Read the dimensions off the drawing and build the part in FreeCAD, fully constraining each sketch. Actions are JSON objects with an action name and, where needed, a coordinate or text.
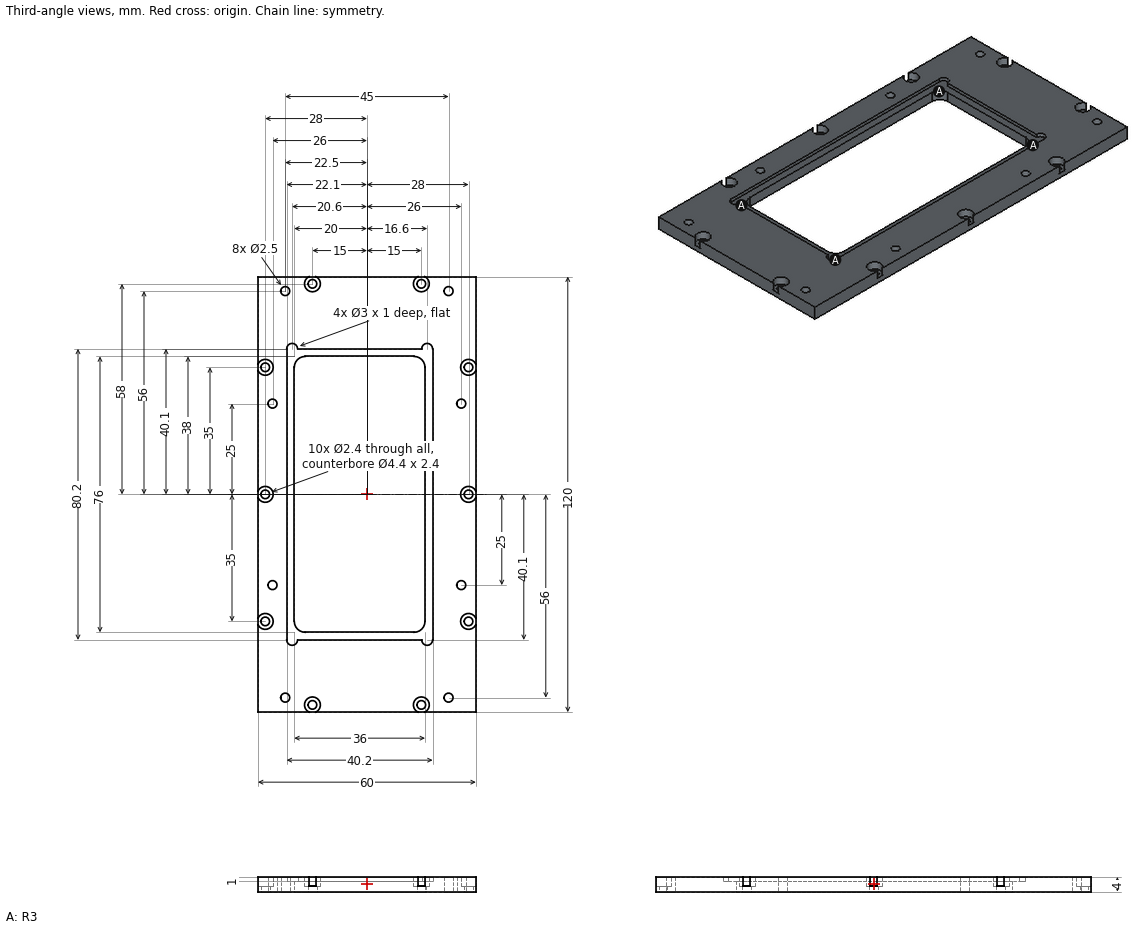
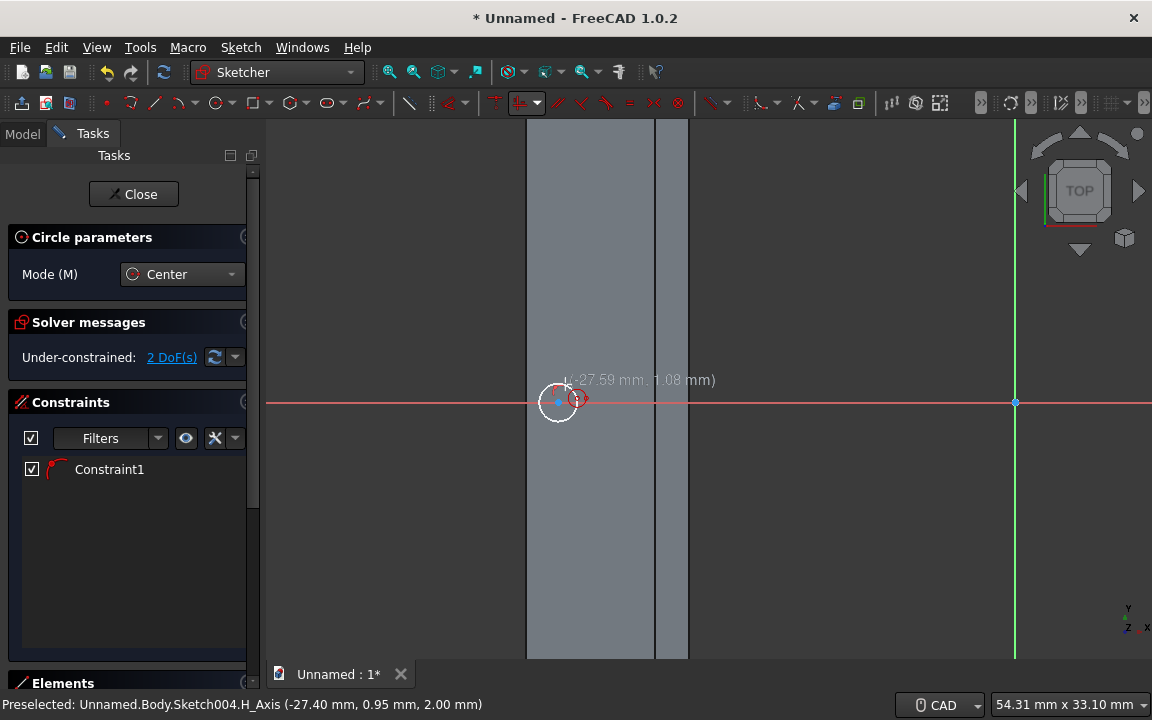
{"action": "scroll", "coordinate": [566, 386], "scroll_direction": "down", "scroll_amount": 9}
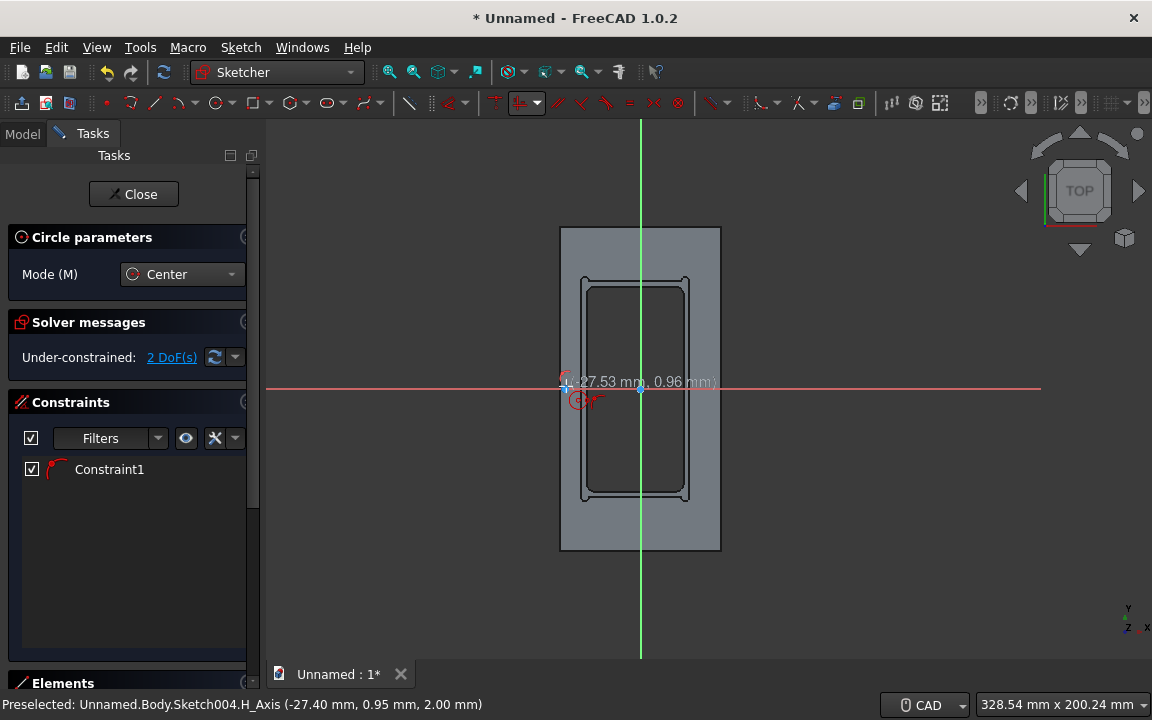
{"action": "scroll", "coordinate": [716, 389], "scroll_direction": "up", "scroll_amount": 10}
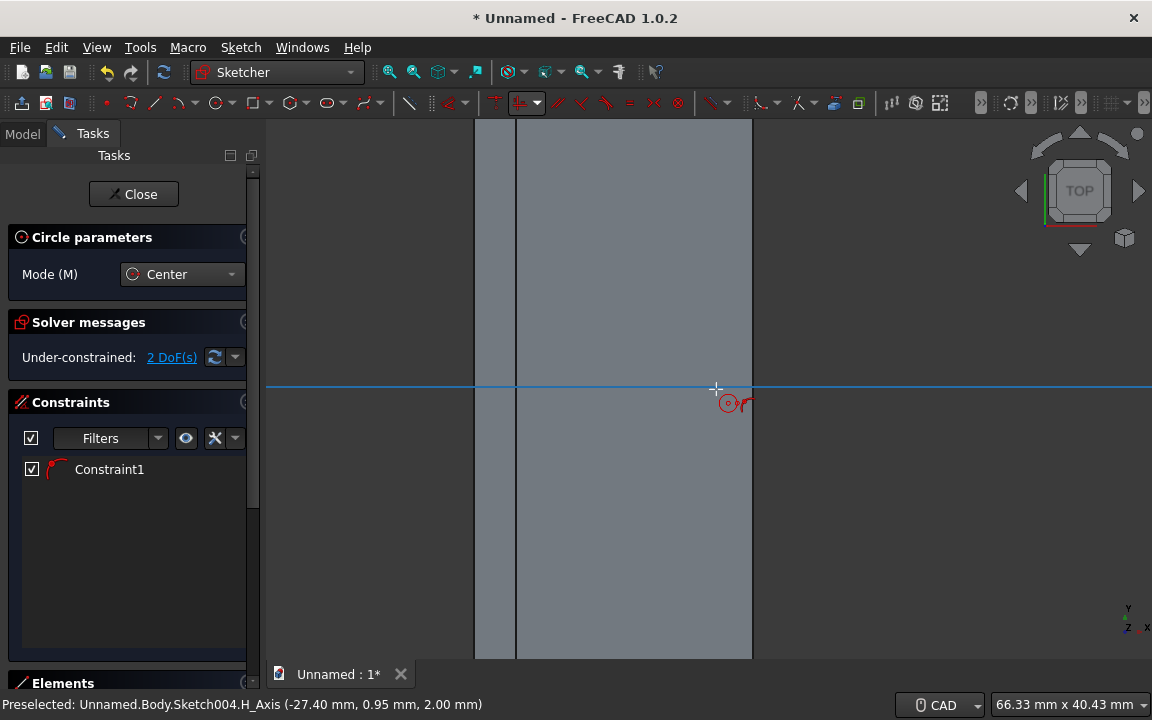
{"action": "scroll", "coordinate": [716, 389], "scroll_direction": "down", "scroll_amount": 10}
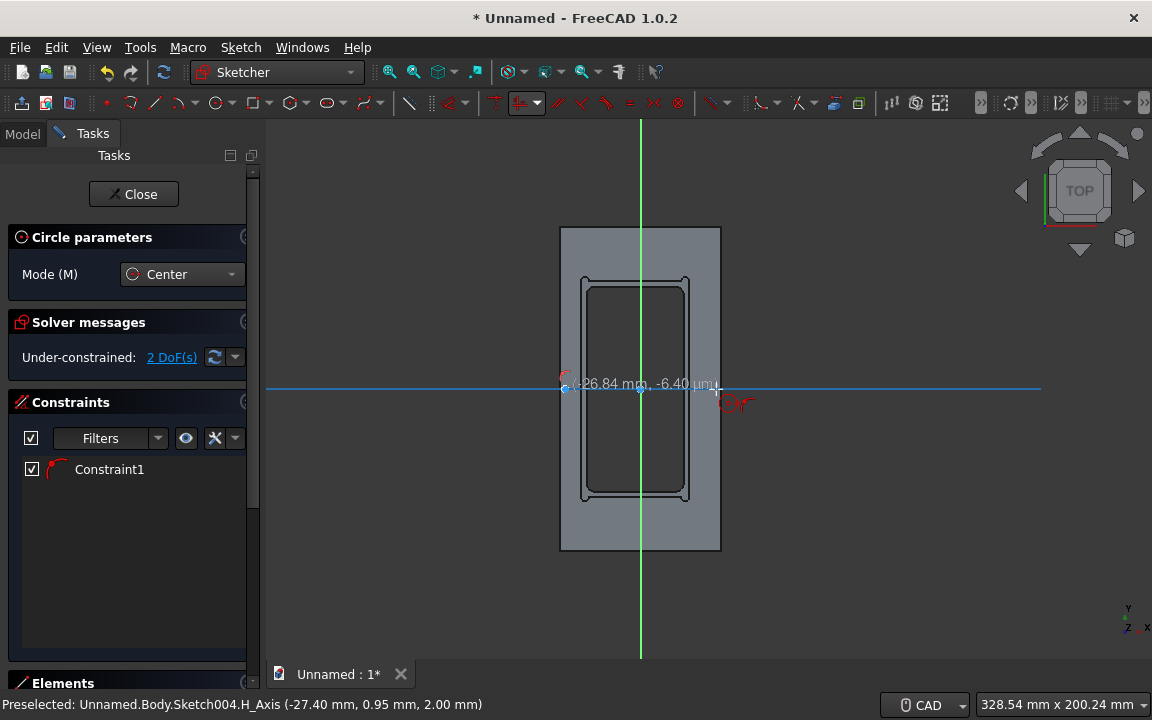
{"action": "left_click", "coordinate": [716, 389]}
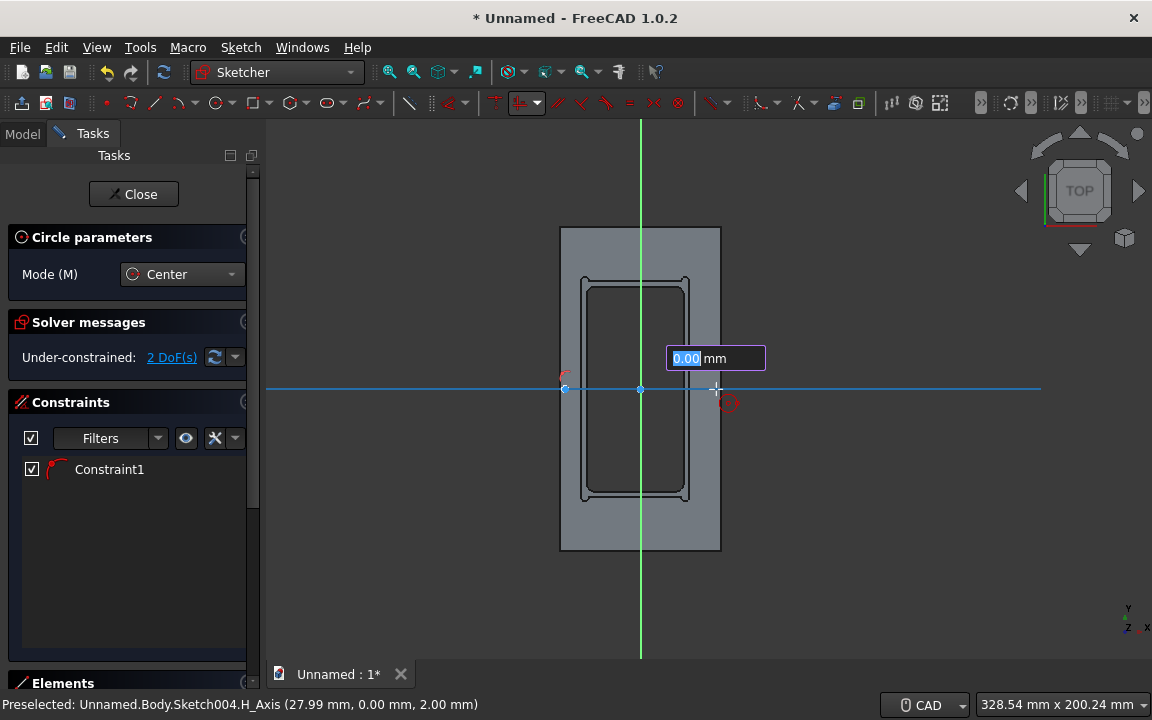
{"action": "scroll", "coordinate": [717, 386], "scroll_direction": "up", "scroll_amount": 9}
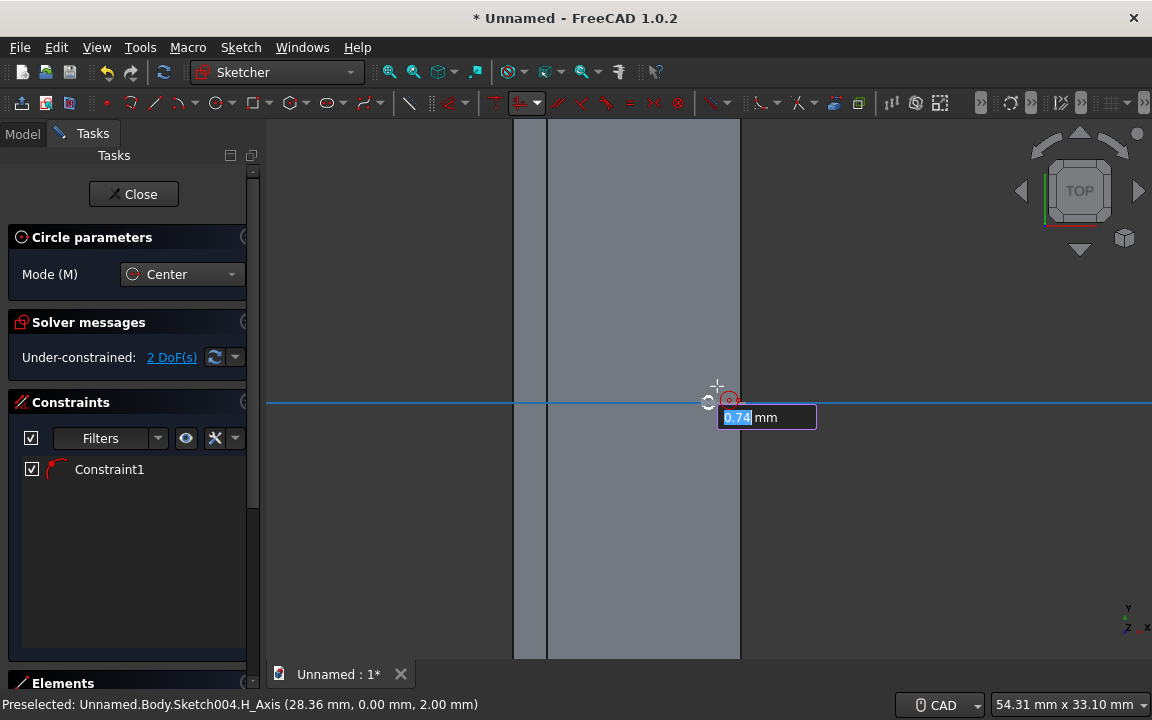
{"action": "left_click", "coordinate": [715, 384]}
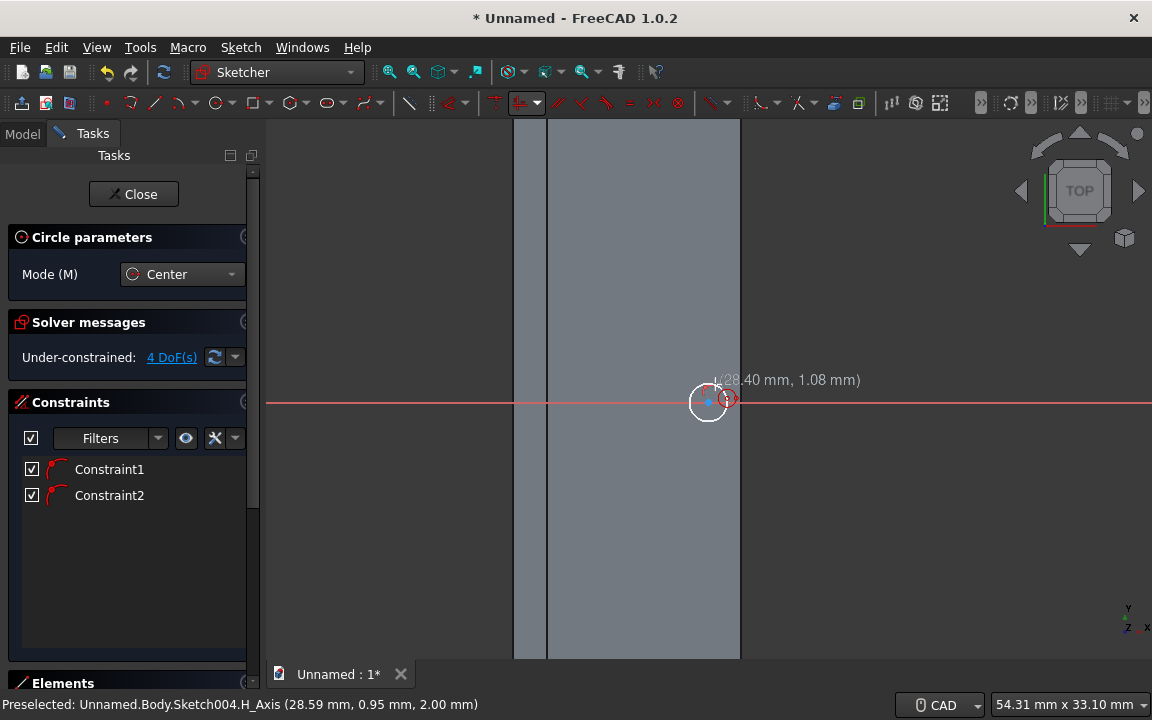
{"action": "scroll", "coordinate": [717, 386], "scroll_direction": "down", "scroll_amount": 9}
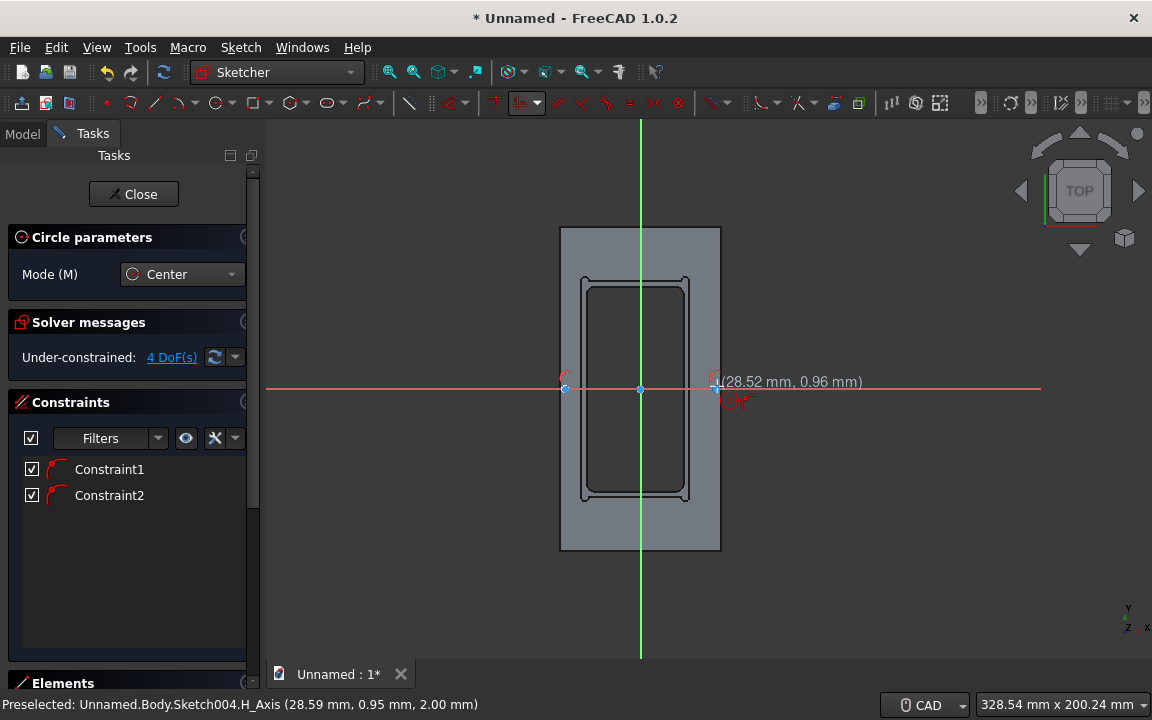
{"action": "scroll", "coordinate": [600, 233], "scroll_direction": "up", "scroll_amount": 10}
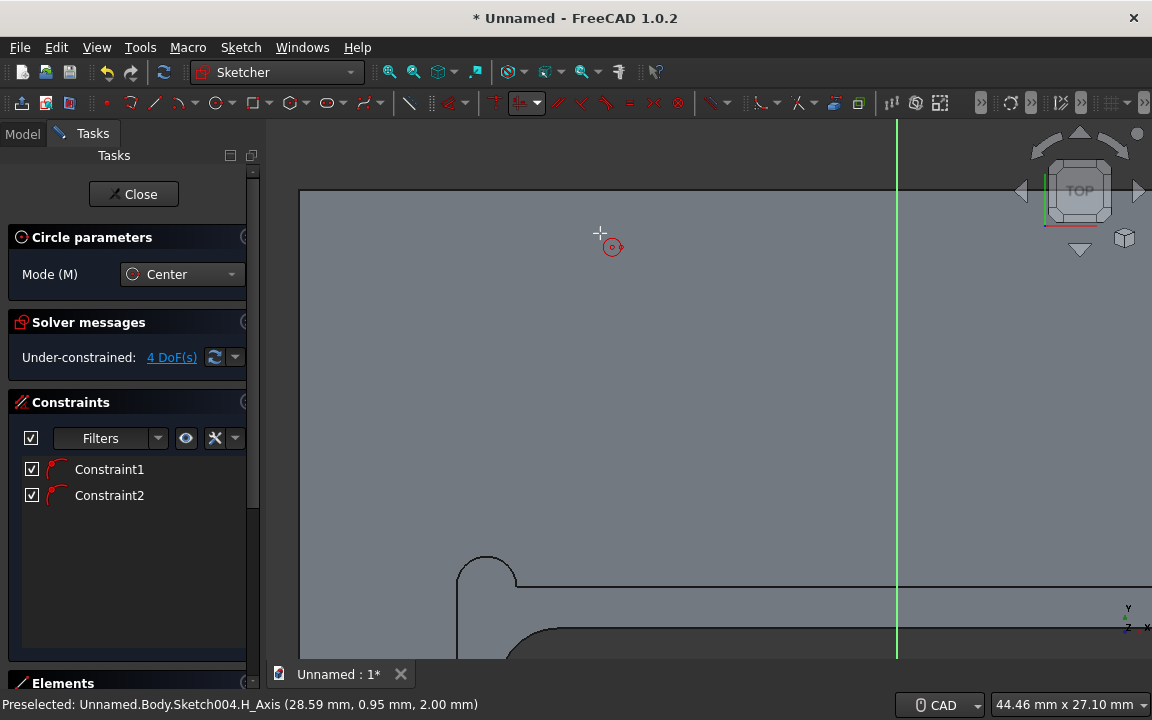
{"action": "scroll", "coordinate": [600, 233], "scroll_direction": "down", "scroll_amount": 10}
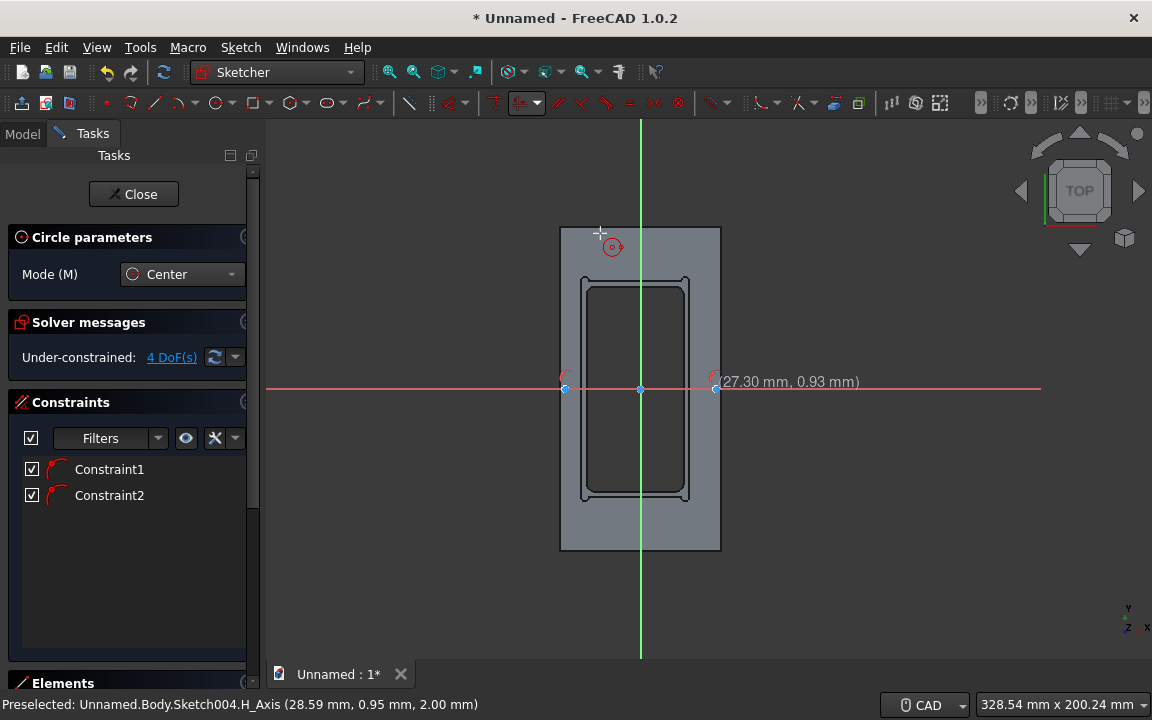
{"action": "left_click", "coordinate": [600, 233]}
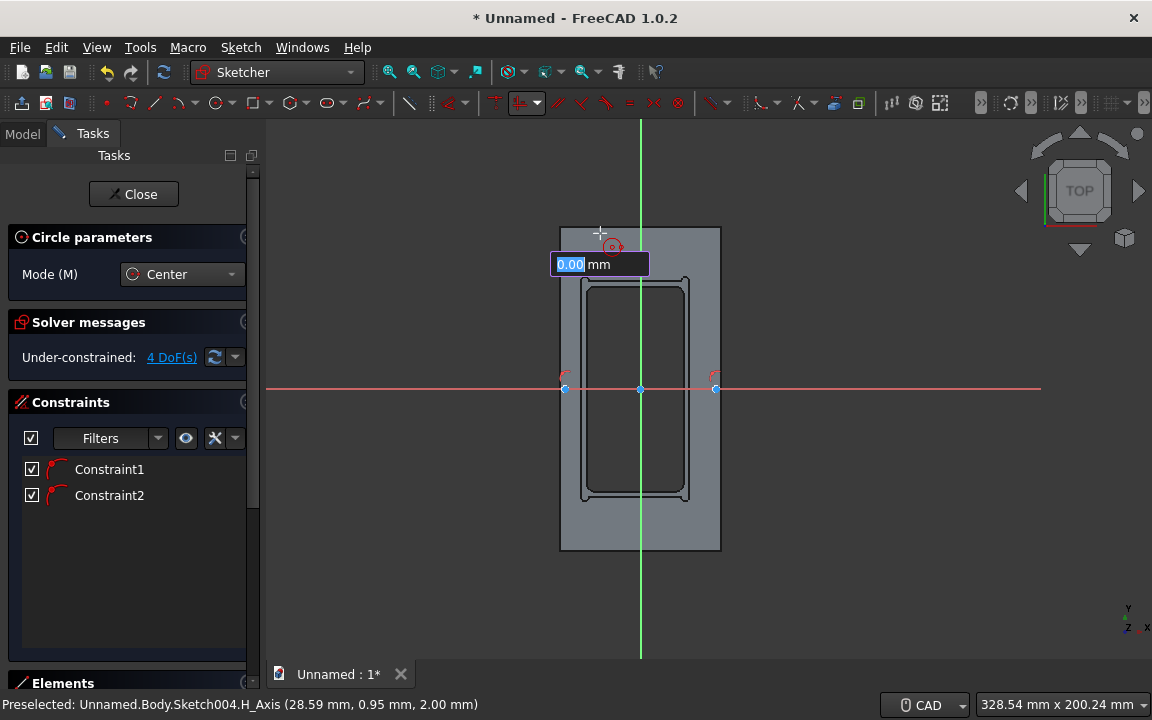
{"action": "scroll", "coordinate": [602, 230], "scroll_direction": "up", "scroll_amount": 8}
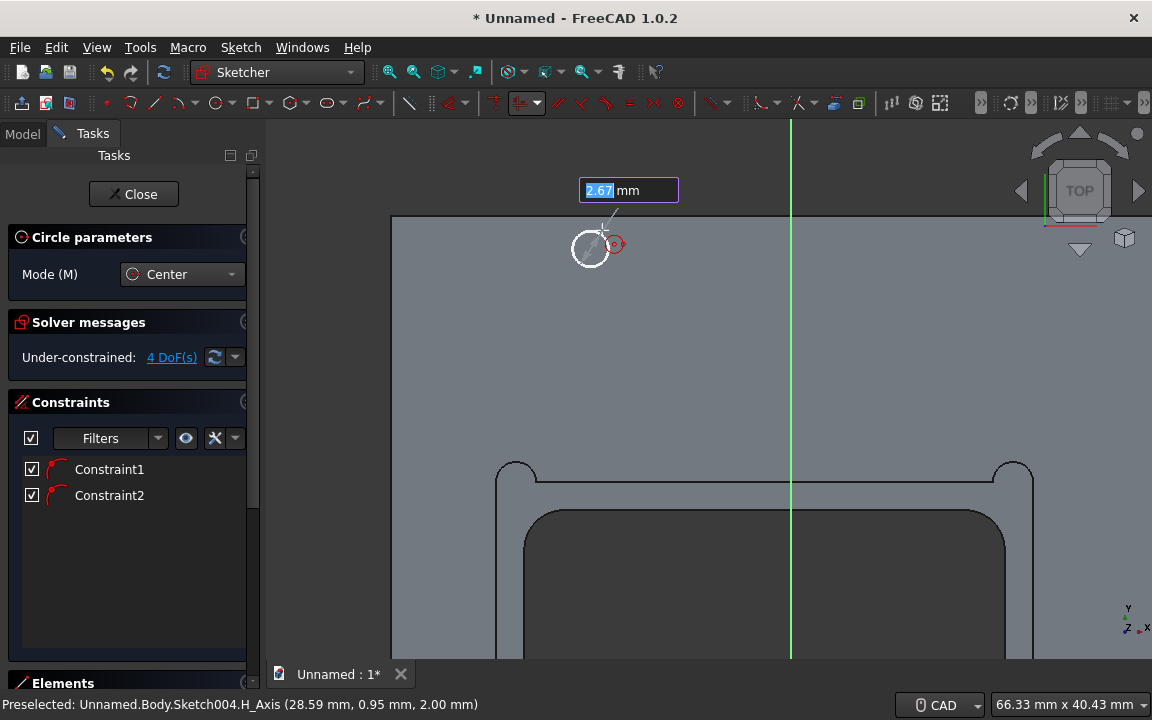
{"action": "left_click", "coordinate": [602, 231]}